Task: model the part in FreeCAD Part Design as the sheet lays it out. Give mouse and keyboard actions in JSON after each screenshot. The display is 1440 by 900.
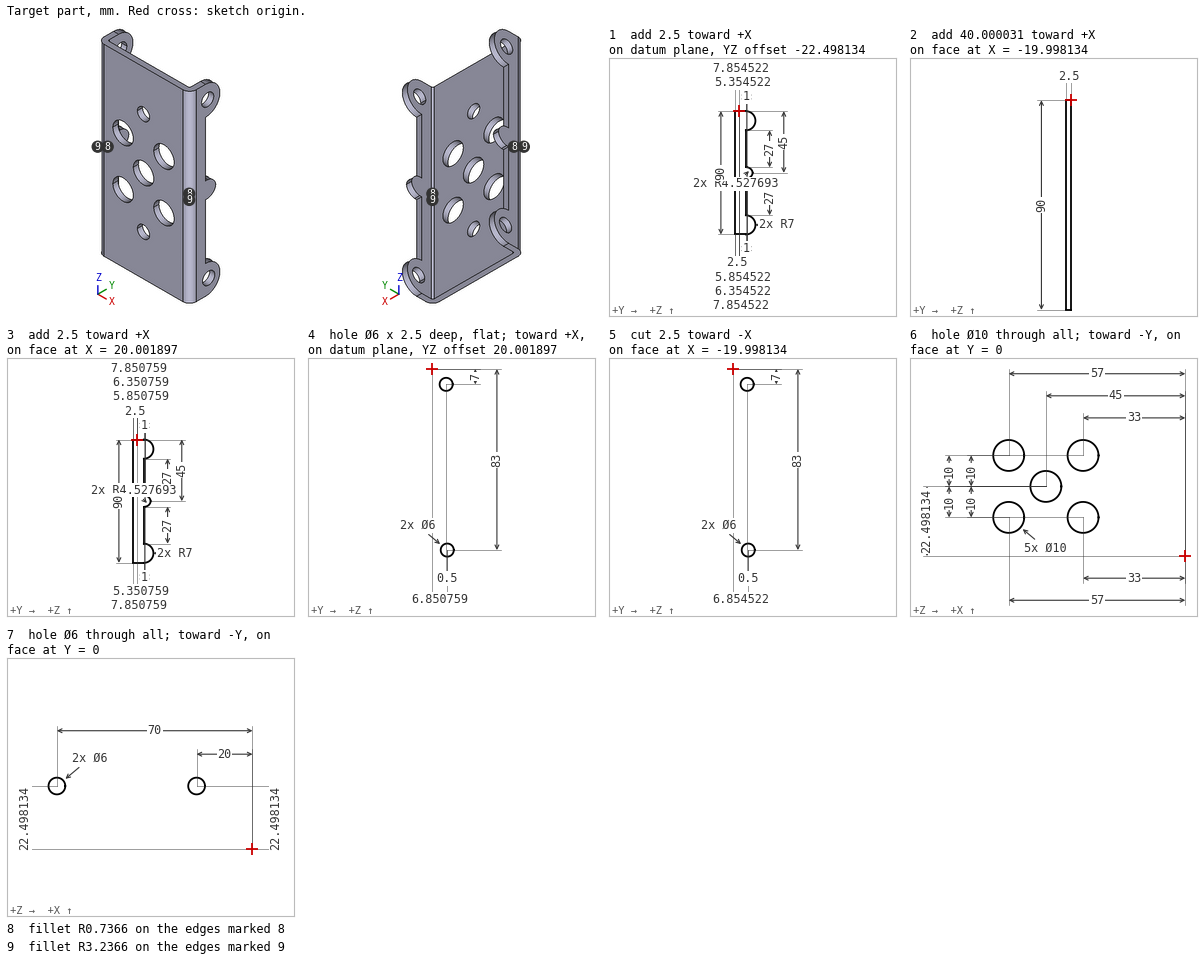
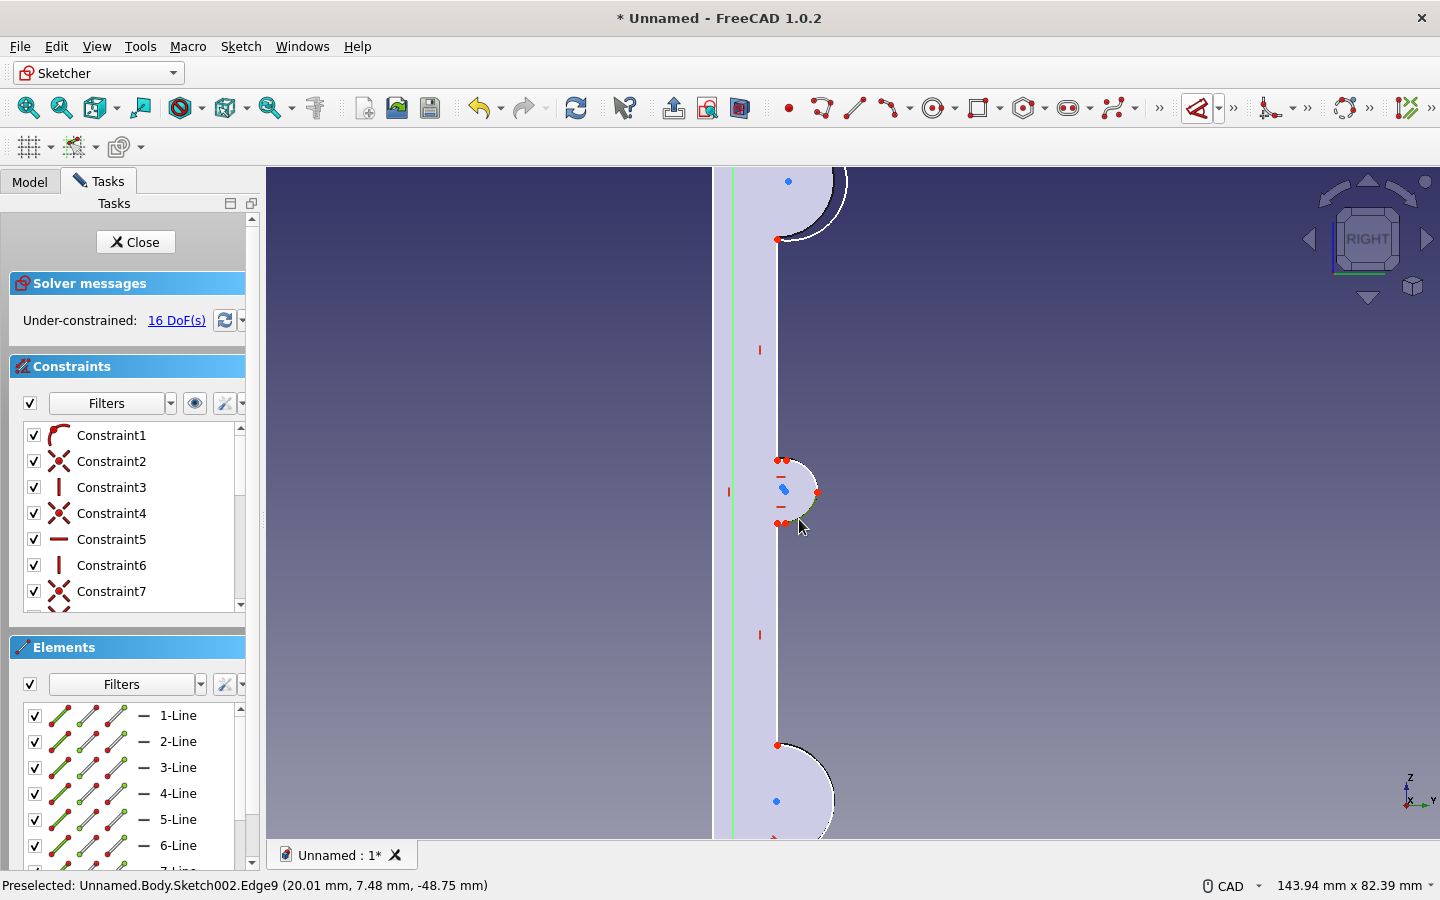
{"action": "left_click", "coordinate": [814, 478]}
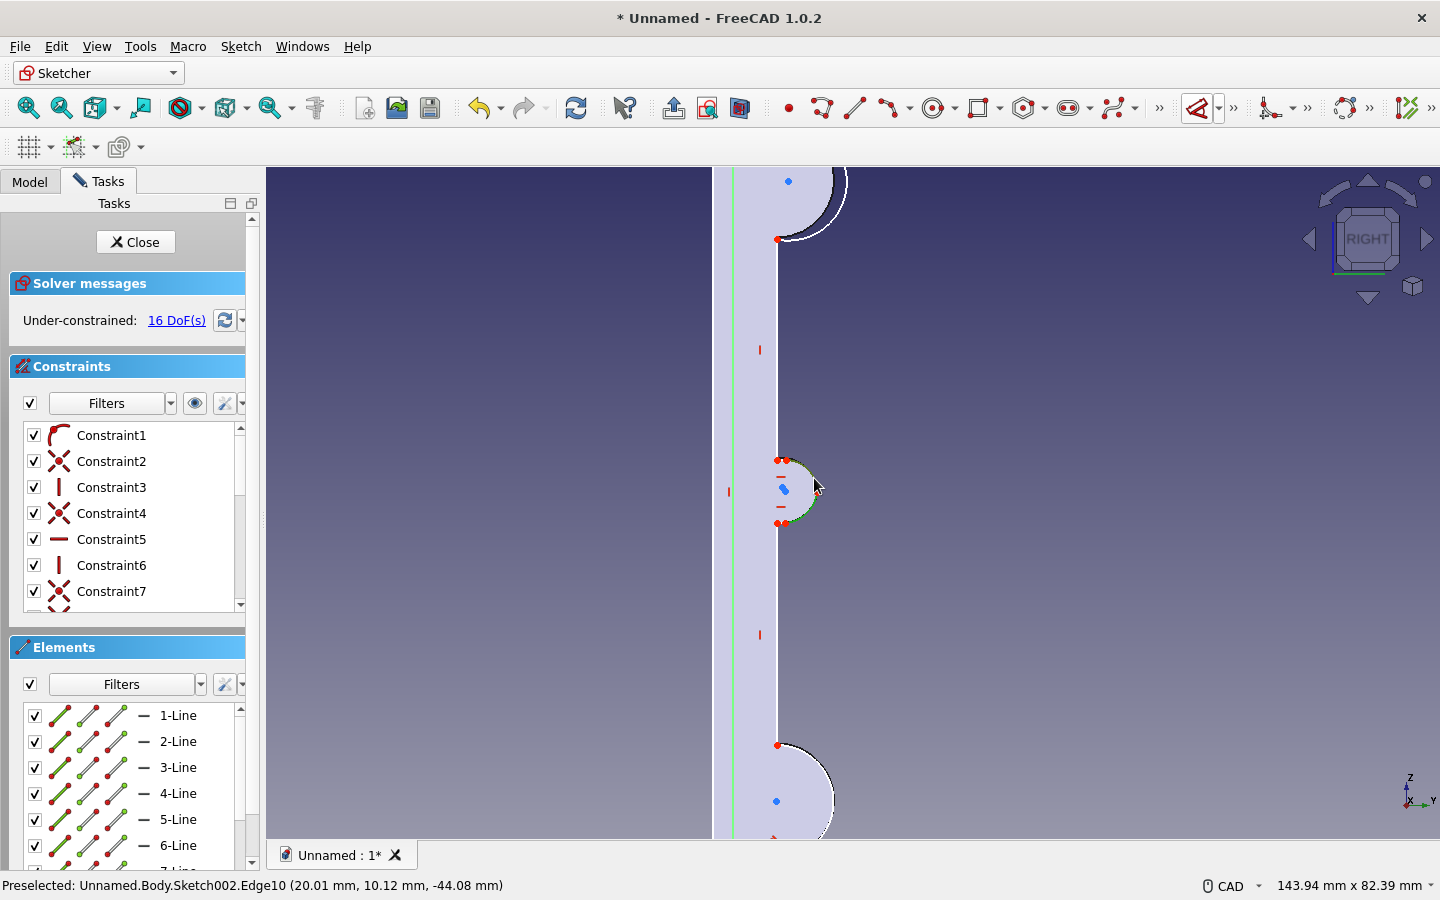
{"action": "key", "text": "e"}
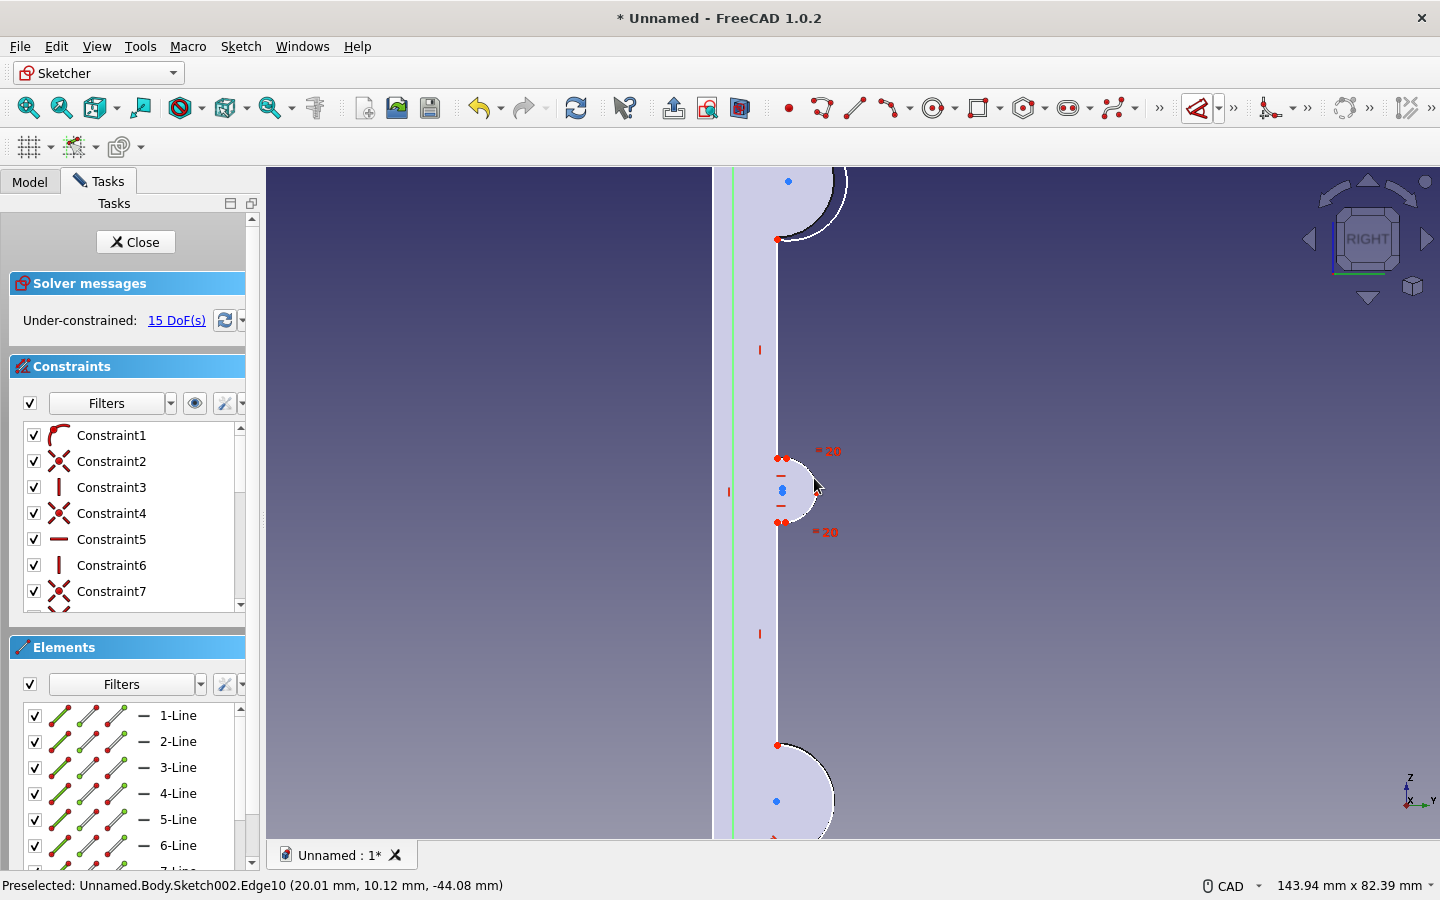
{"action": "left_click", "coordinate": [823, 769]}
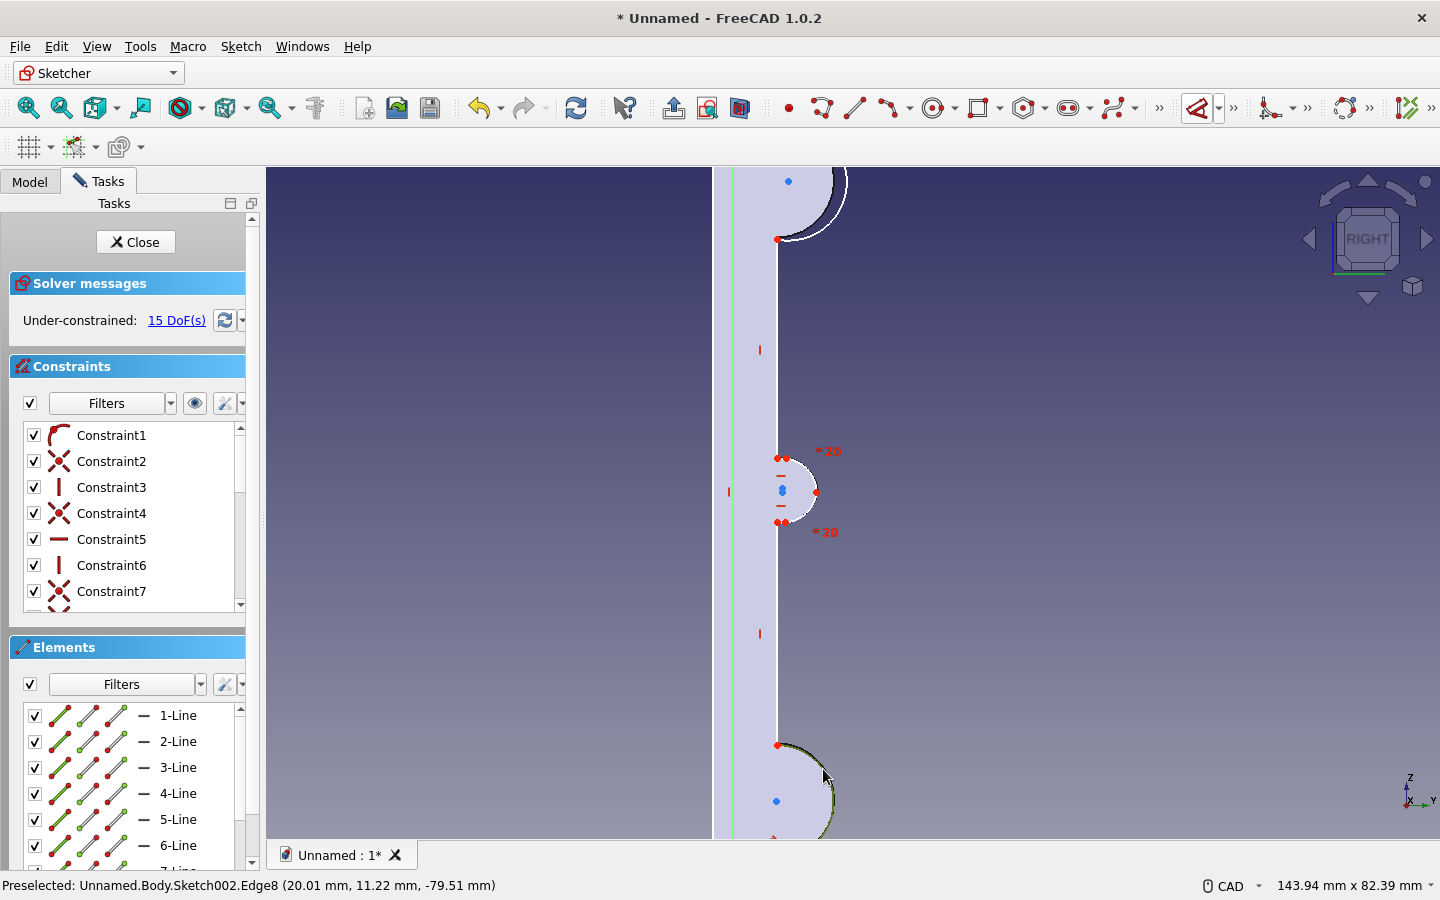
{"action": "left_click", "coordinate": [831, 222]}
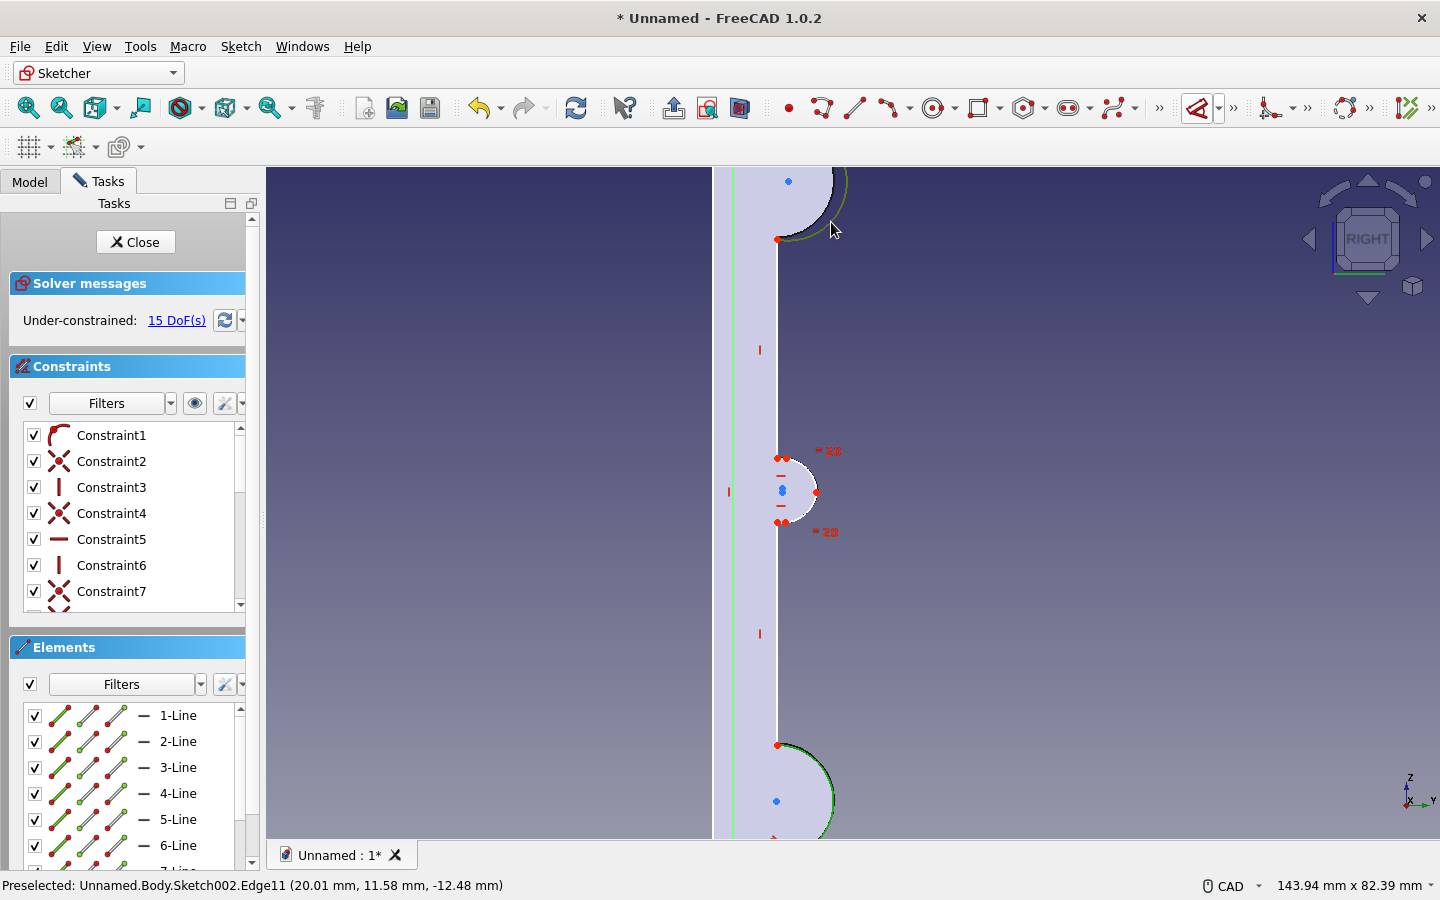
{"action": "key", "text": "e"}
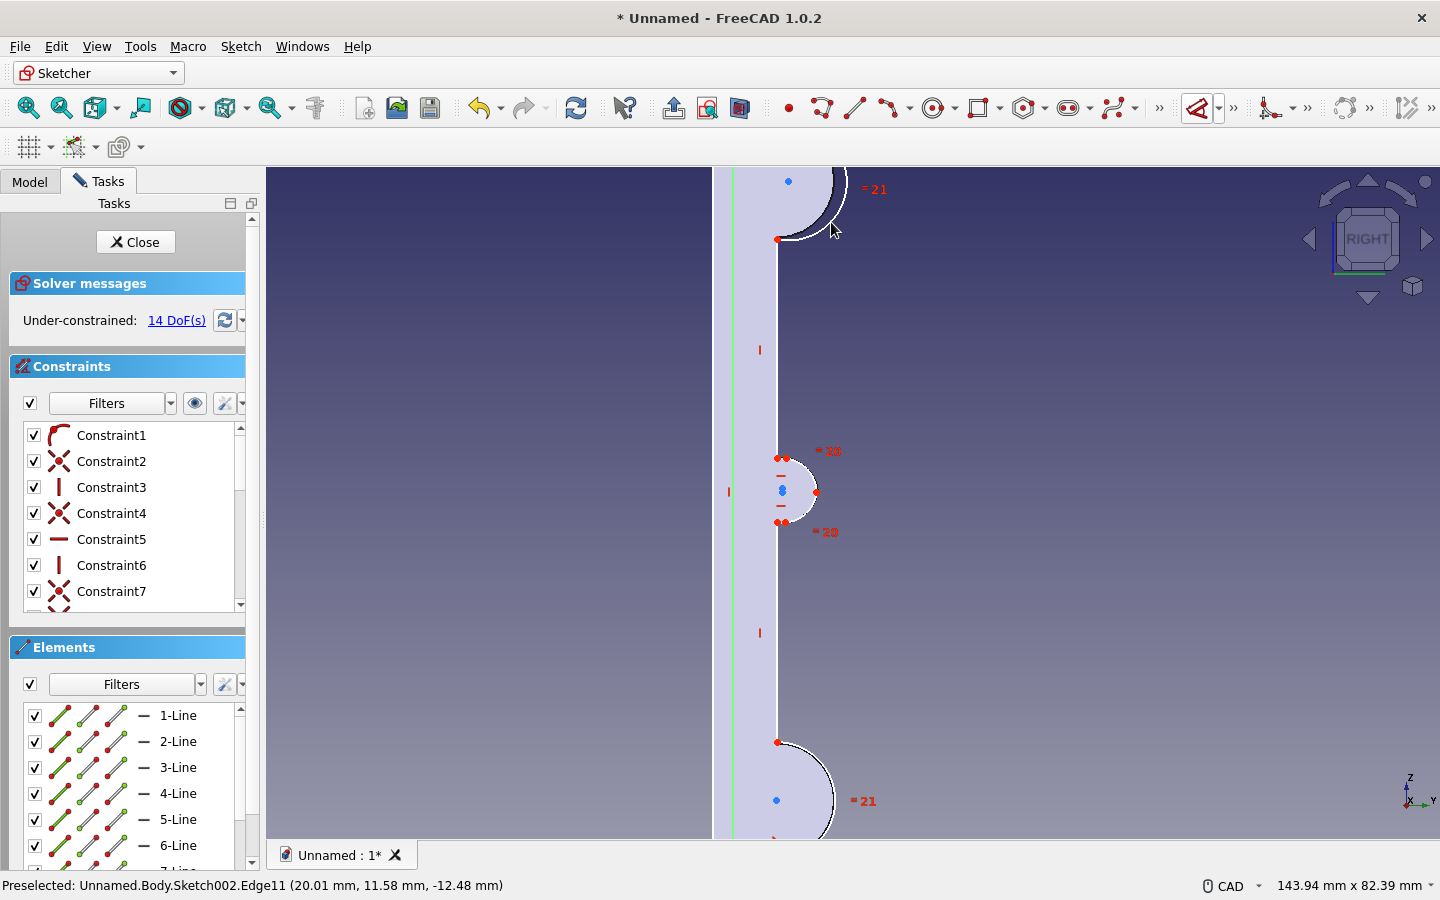
{"action": "left_click", "coordinate": [824, 767]}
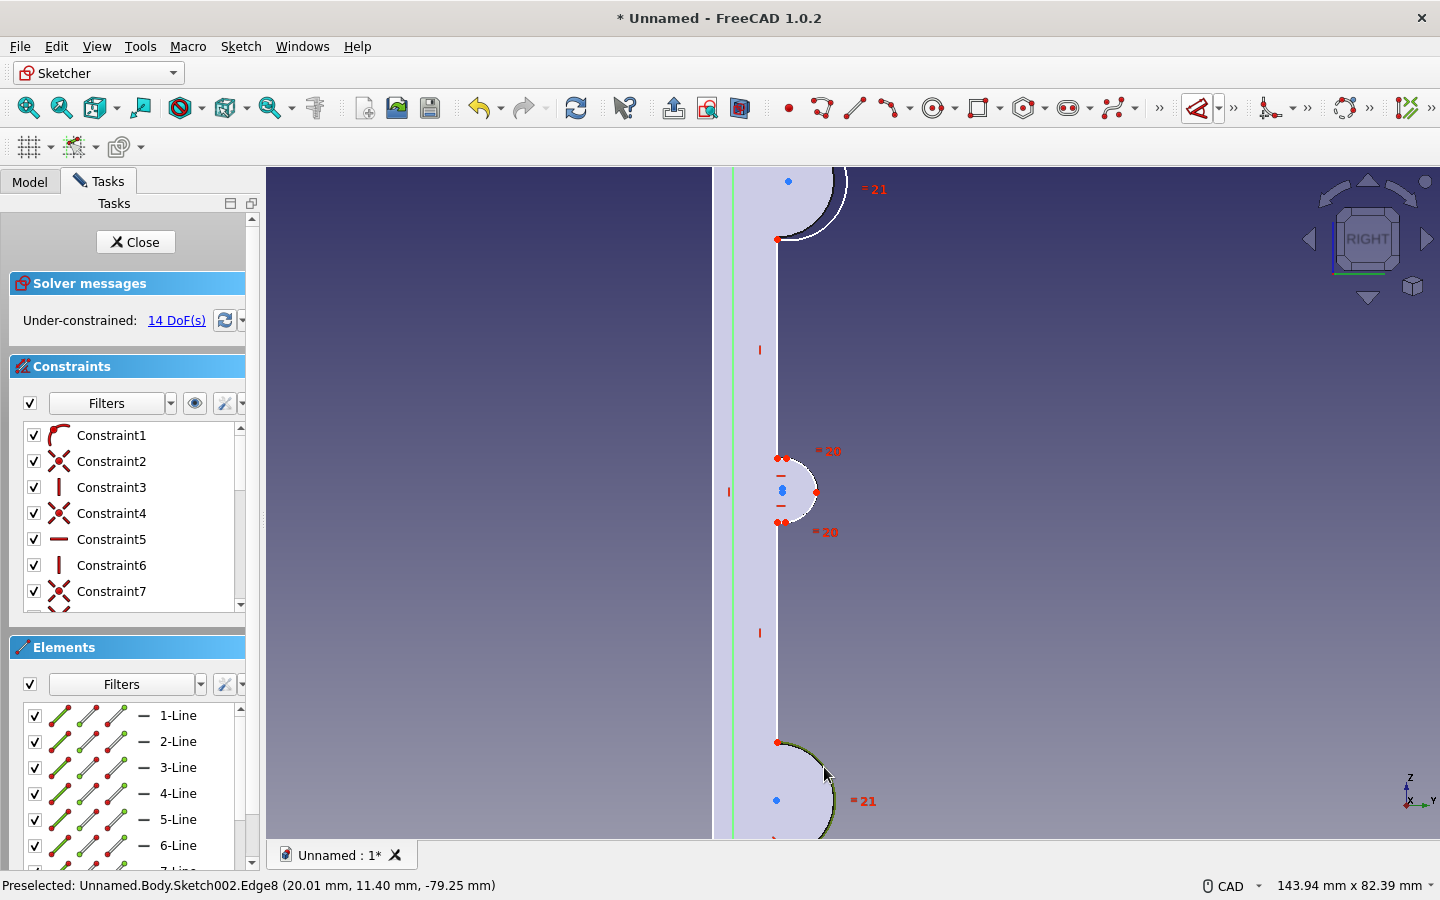
{"action": "left_click", "coordinate": [1218, 108]}